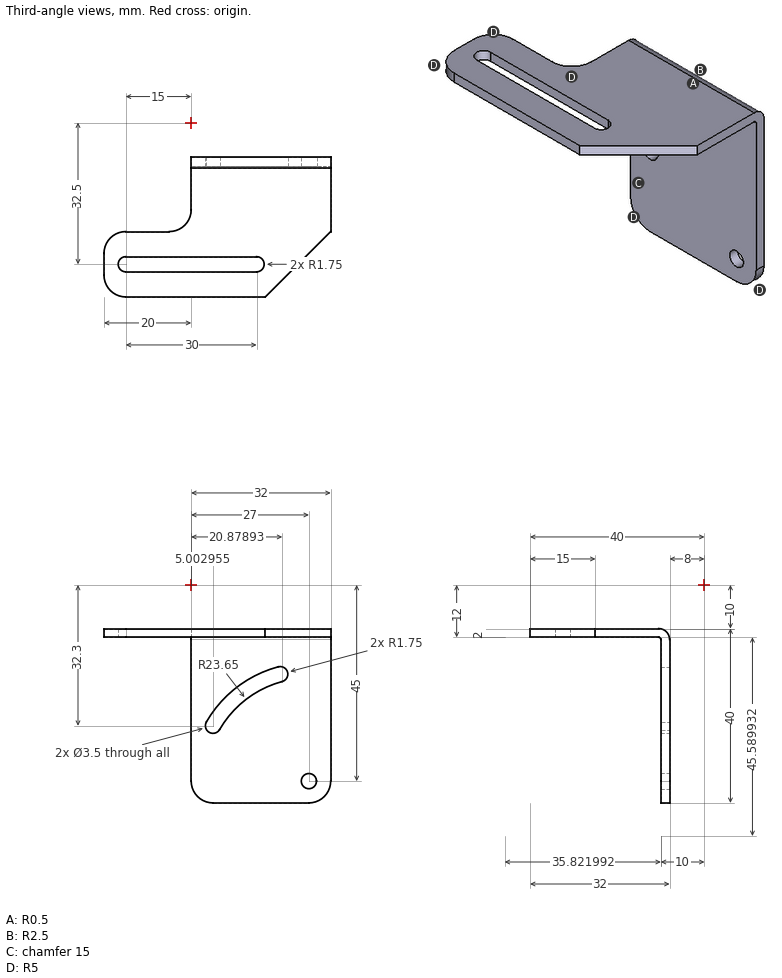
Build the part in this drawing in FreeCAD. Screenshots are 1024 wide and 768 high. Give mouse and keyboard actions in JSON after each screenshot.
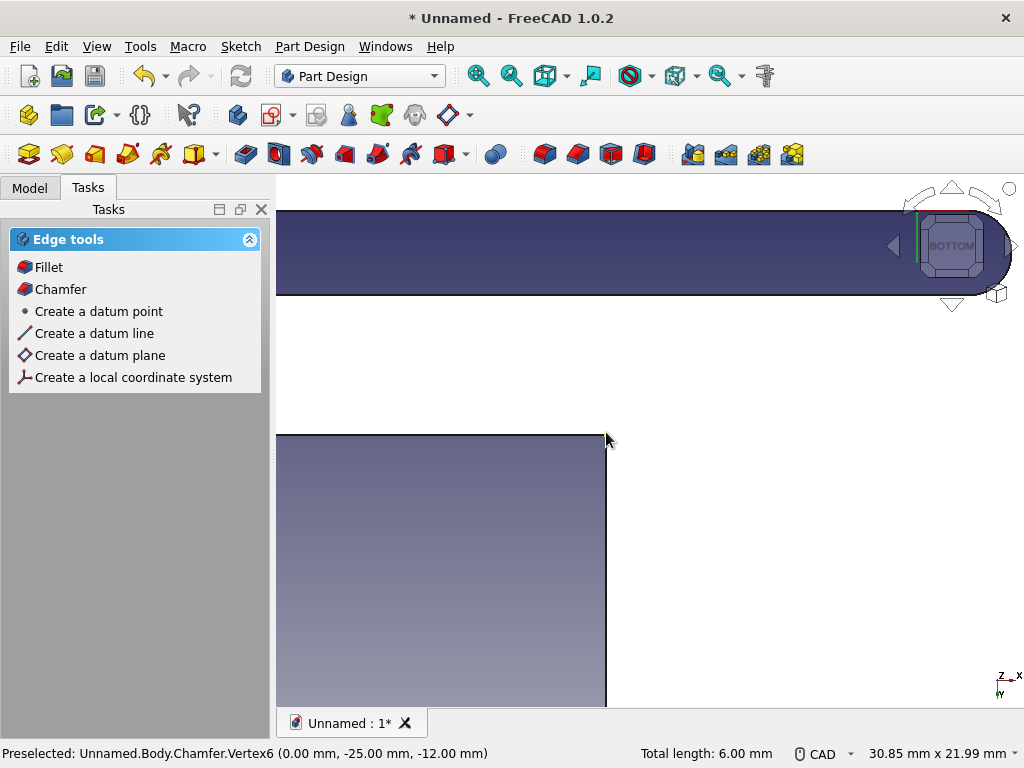
{"action": "key", "text": "v f"}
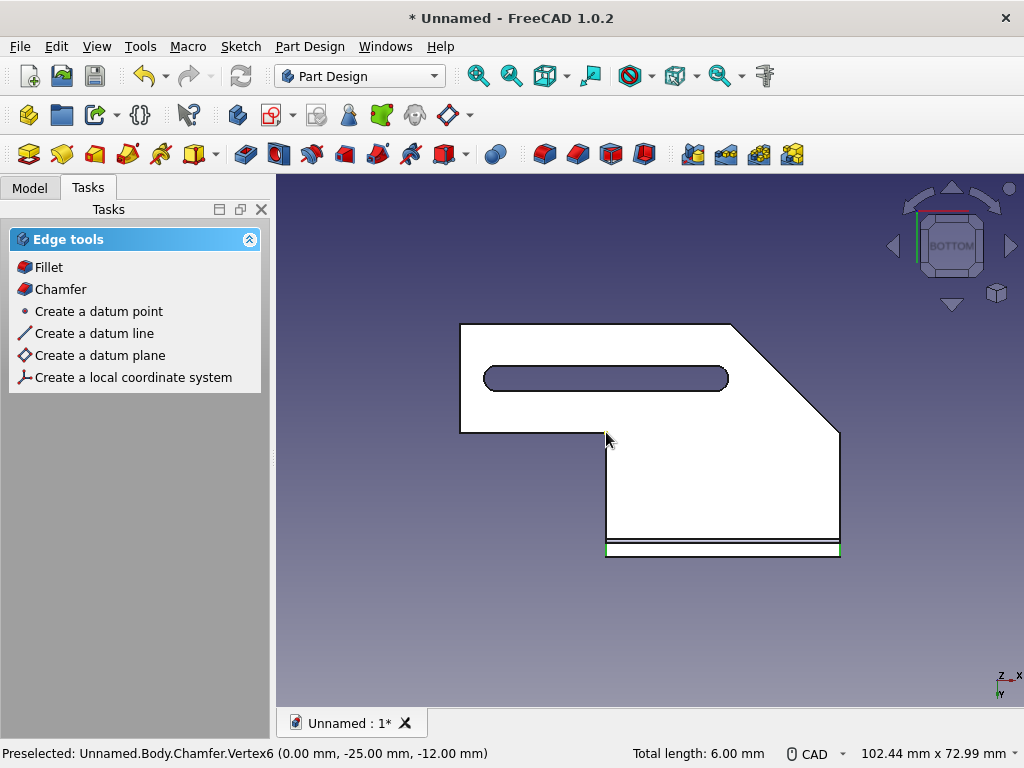
{"action": "key", "text": "4"}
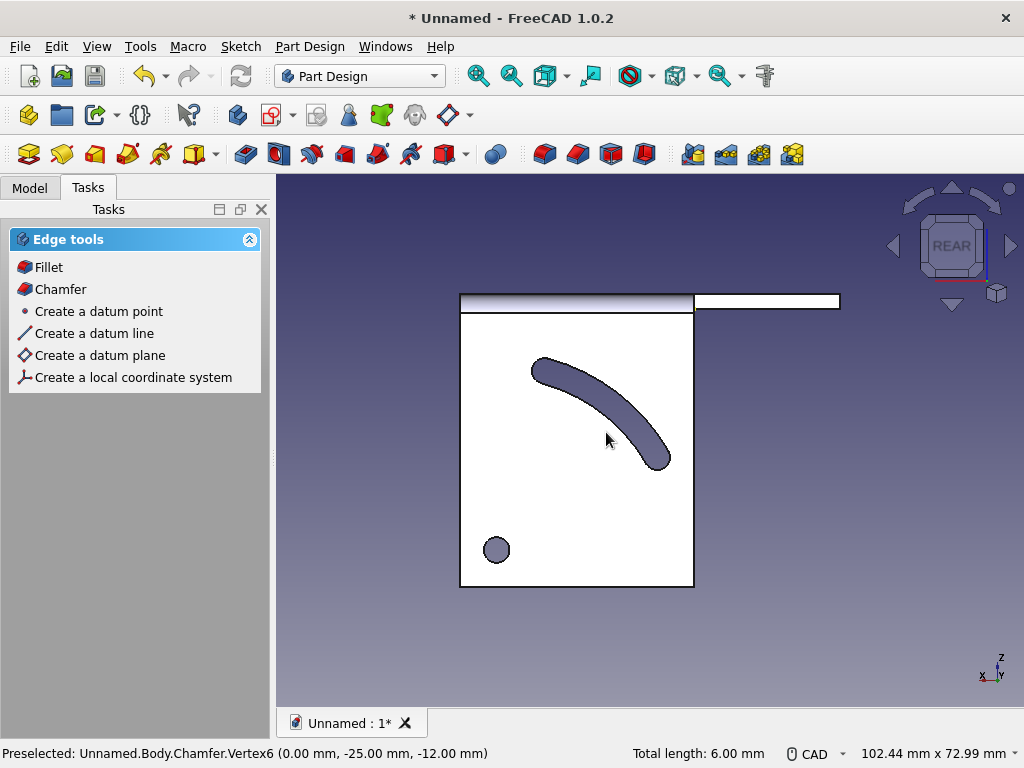
{"action": "left_click", "coordinate": [840, 301], "text": "ctrl"}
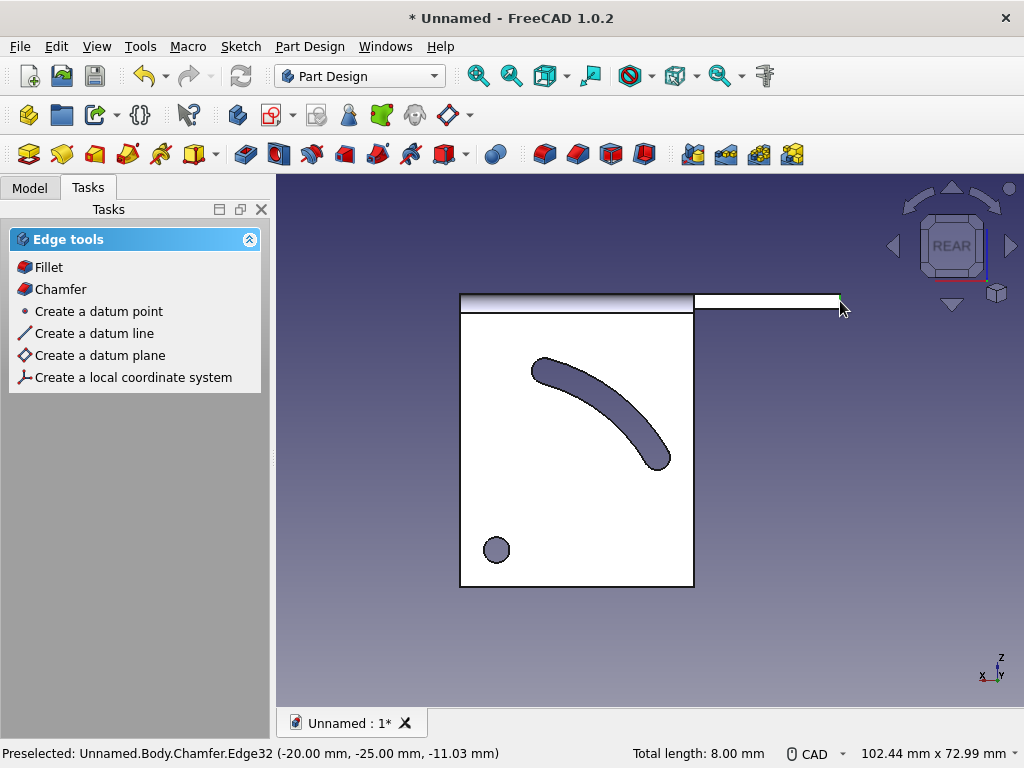
{"action": "scroll", "coordinate": [694, 301], "scroll_direction": "up", "scroll_amount": 6}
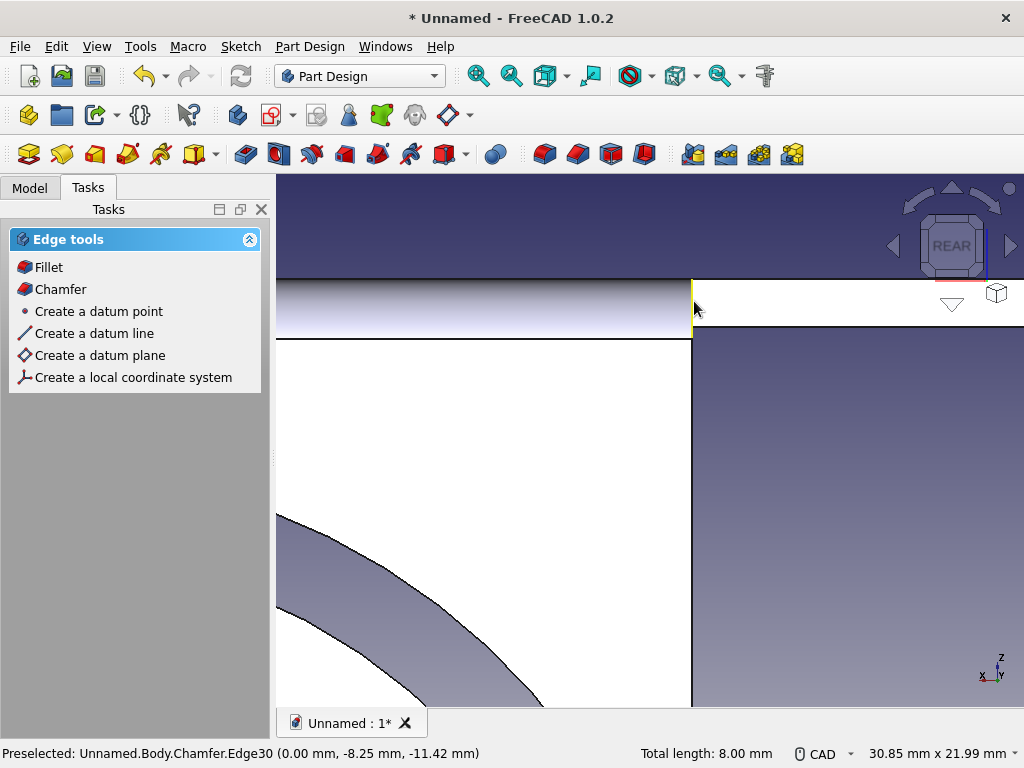
{"action": "key", "text": "v f"}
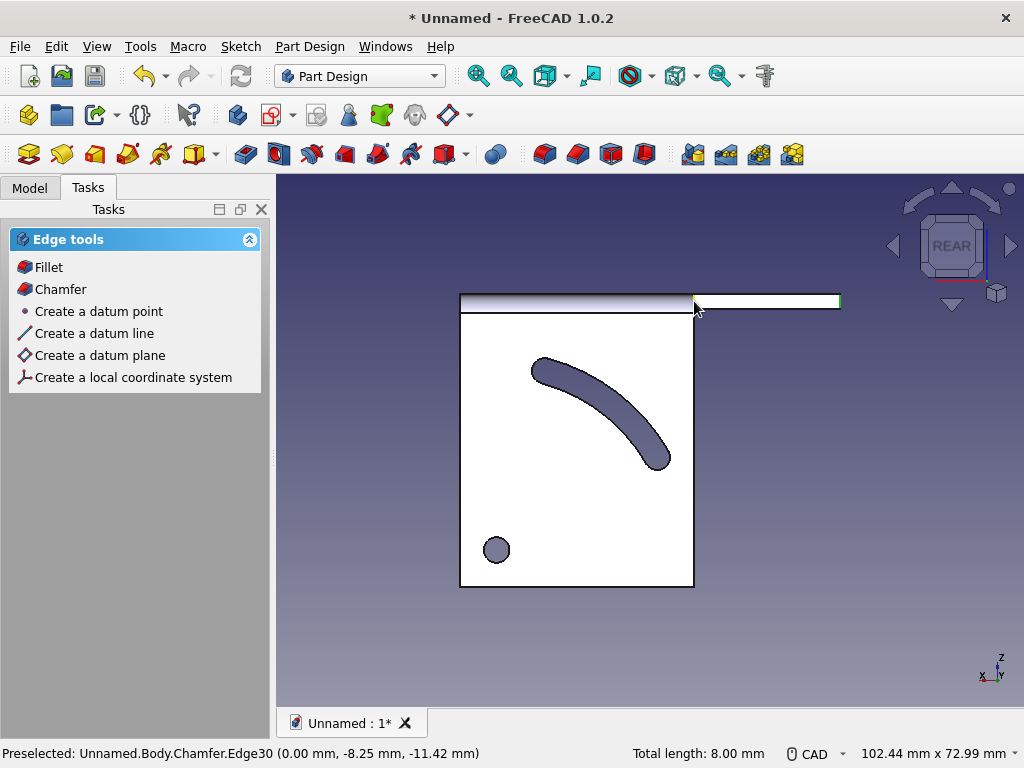
{"action": "key", "text": "6"}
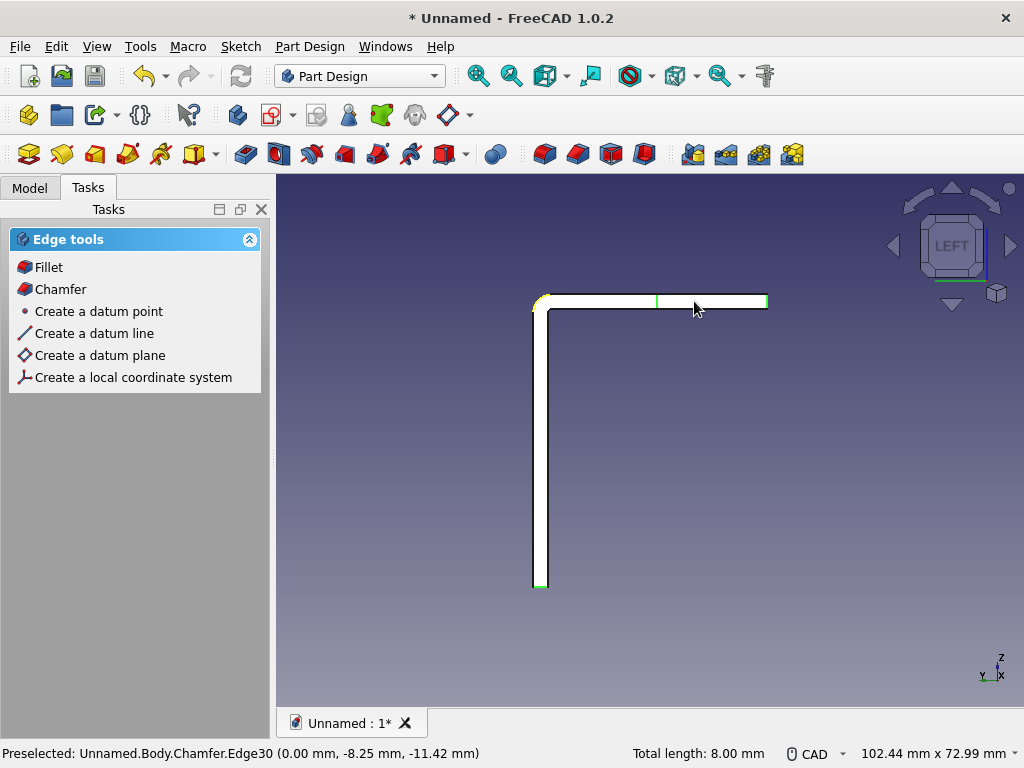
{"action": "scroll", "coordinate": [657, 301], "scroll_direction": "up", "scroll_amount": 6}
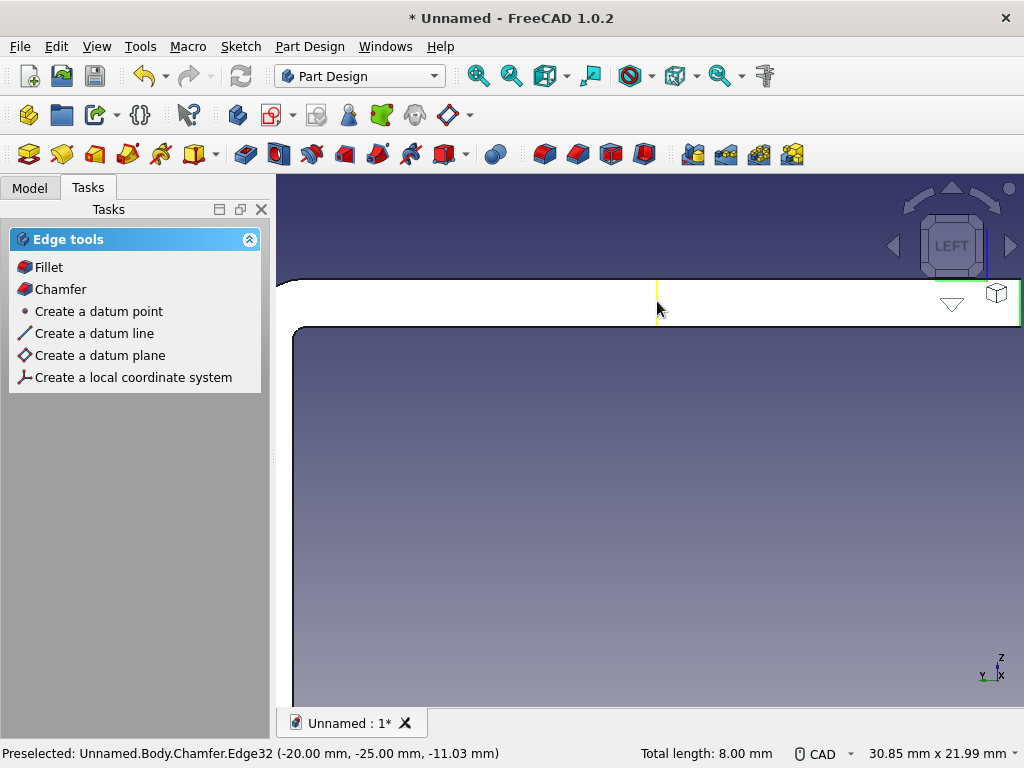
{"action": "left_click", "coordinate": [479, 76]}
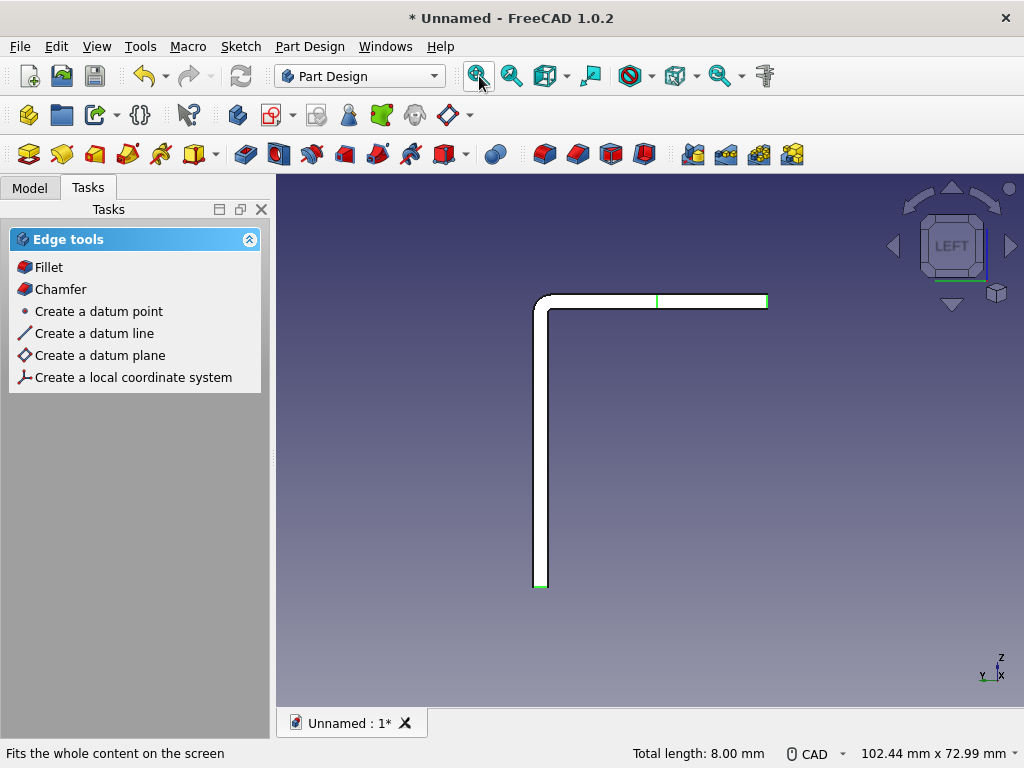
{"action": "key", "text": "v 3"}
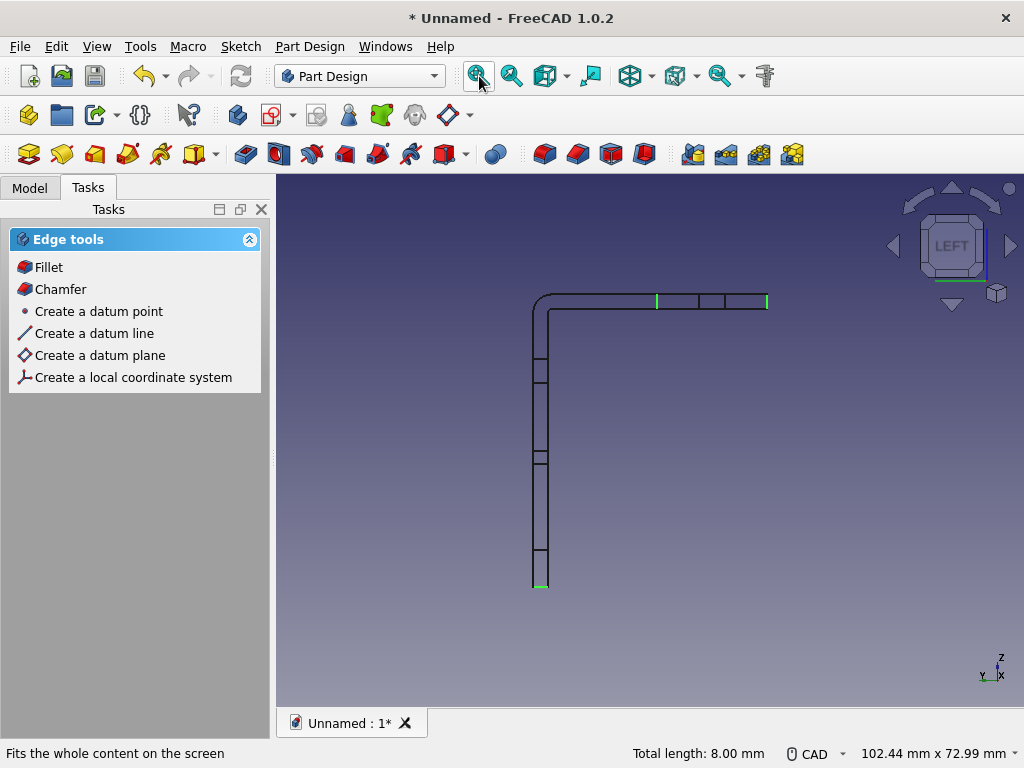
{"action": "key", "text": "0"}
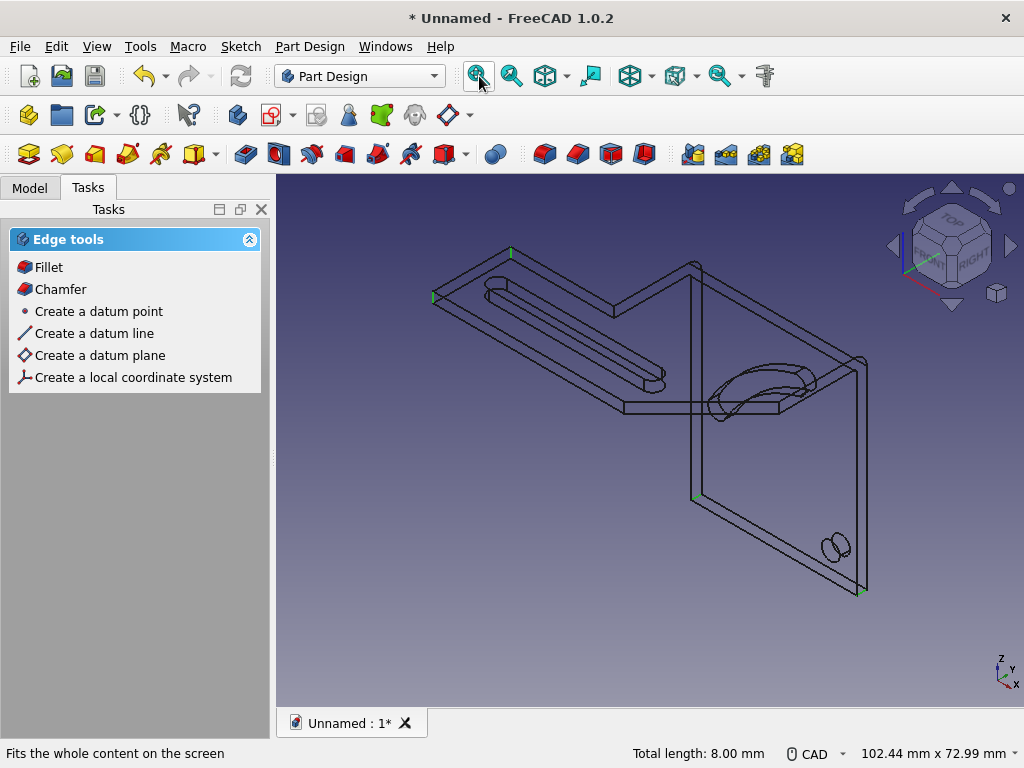
{"action": "left_click", "coordinate": [614, 313], "text": "ctrl"}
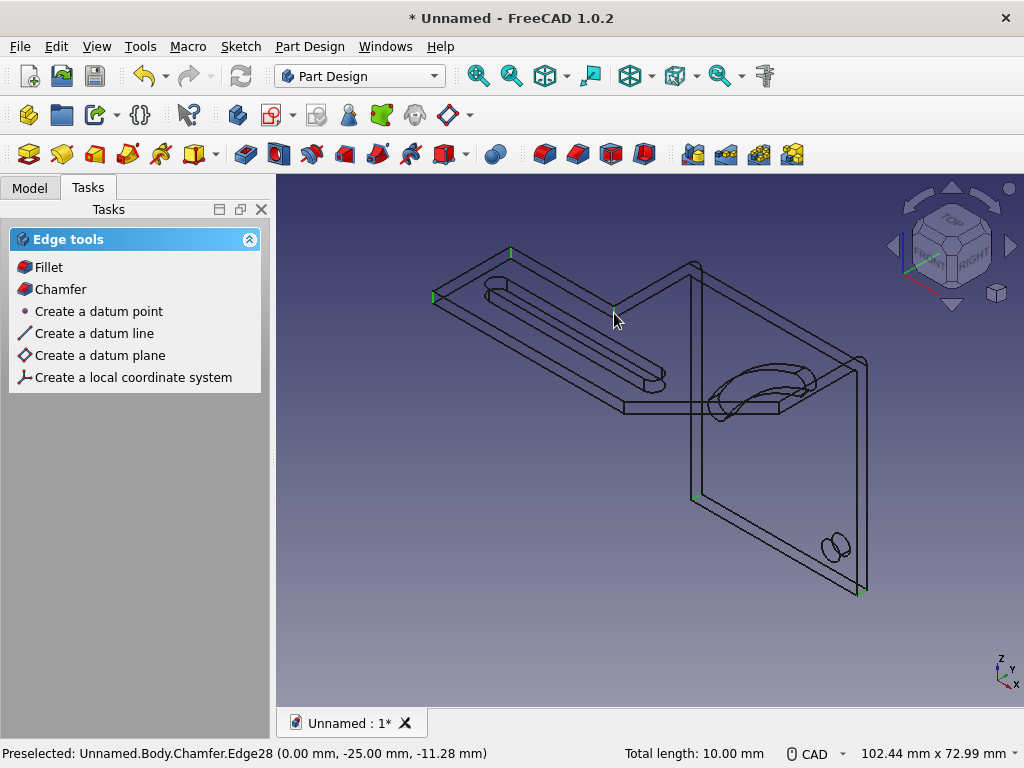
{"action": "key", "text": "v 1"}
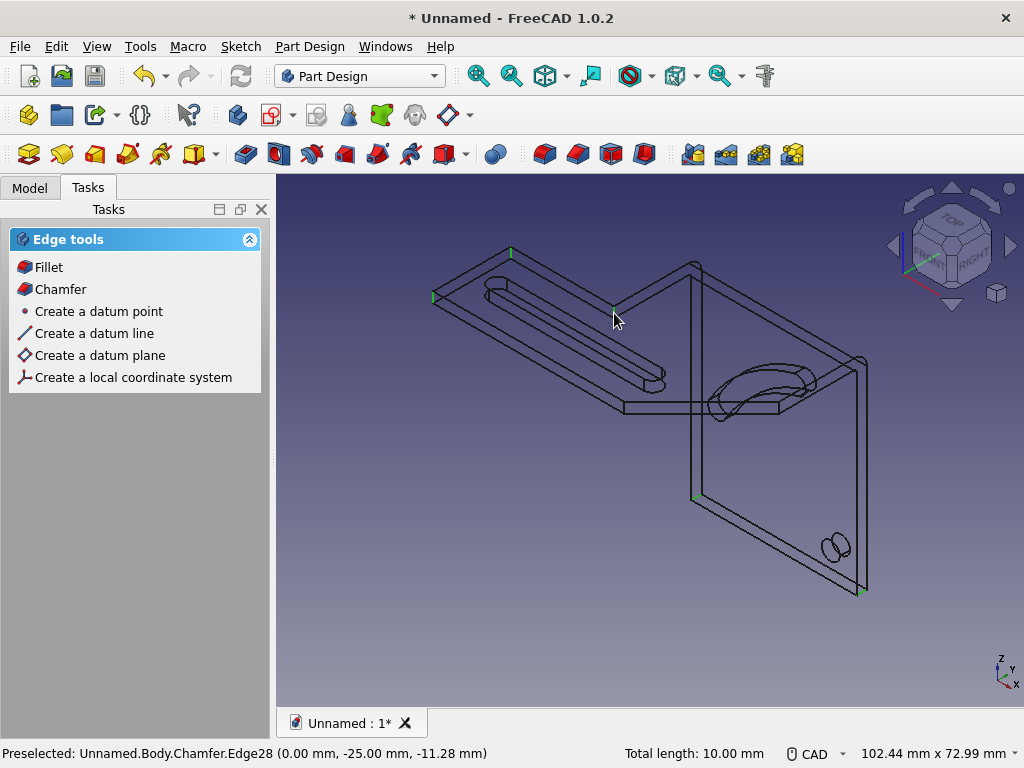
{"action": "left_click", "coordinate": [545, 154]}